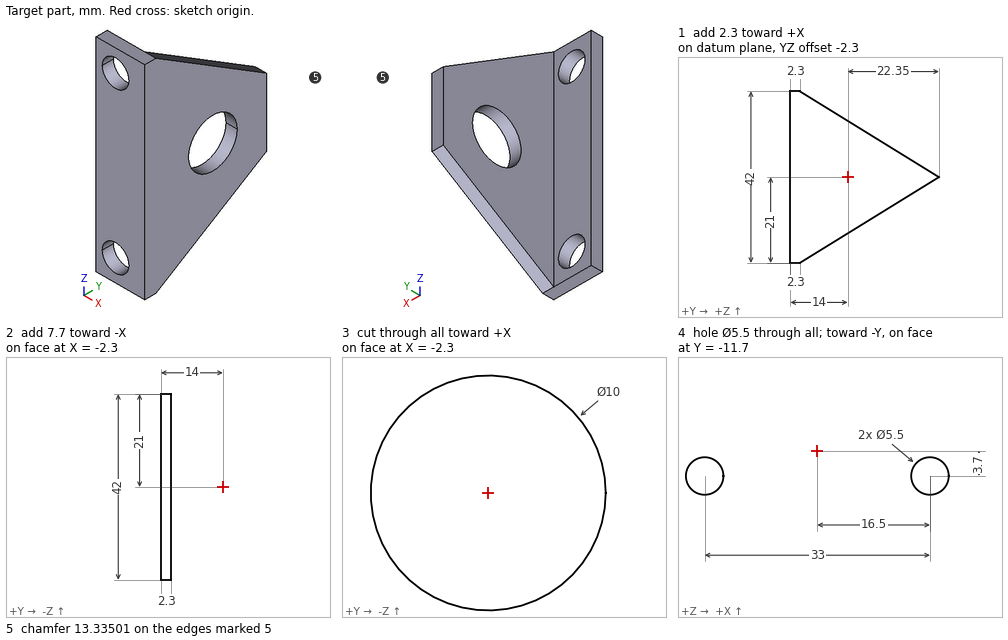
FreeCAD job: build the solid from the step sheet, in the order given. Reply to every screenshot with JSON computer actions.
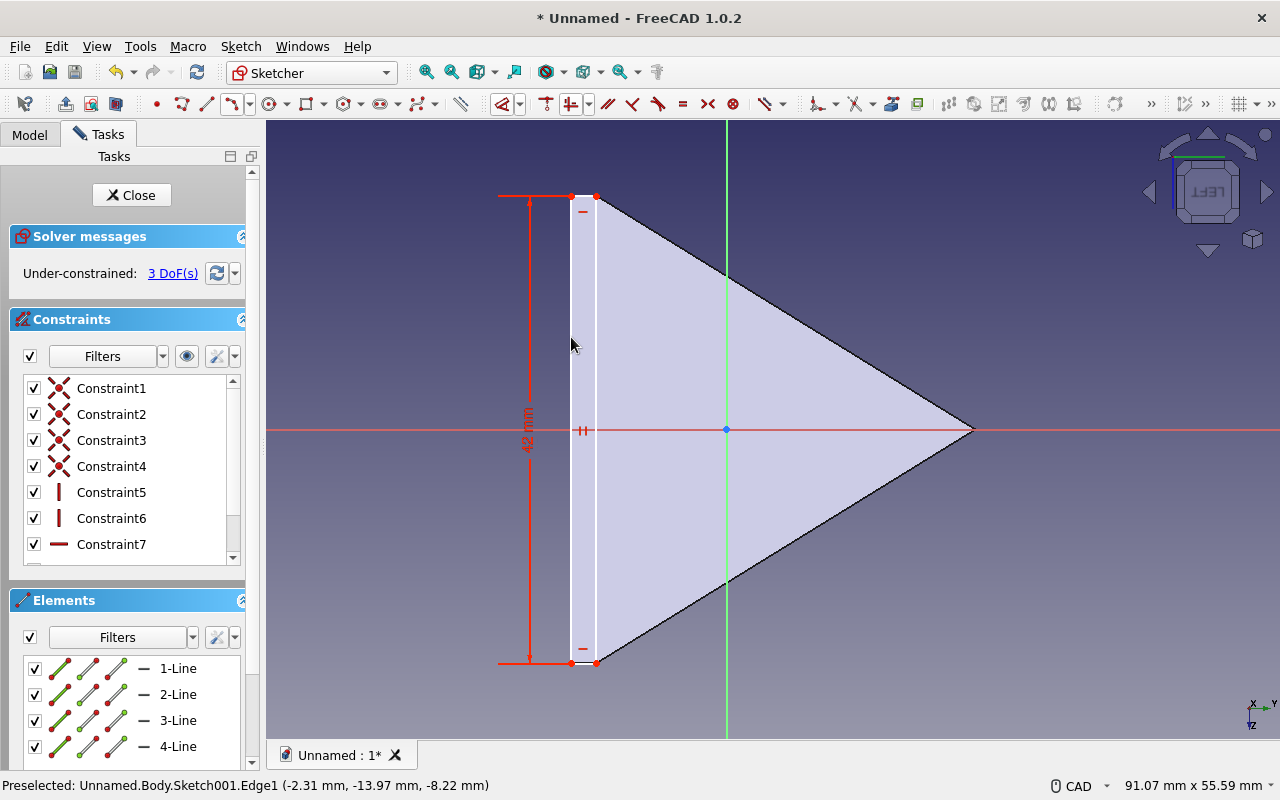
{"action": "scroll", "coordinate": [581, 664], "scroll_direction": "up", "scroll_amount": 3}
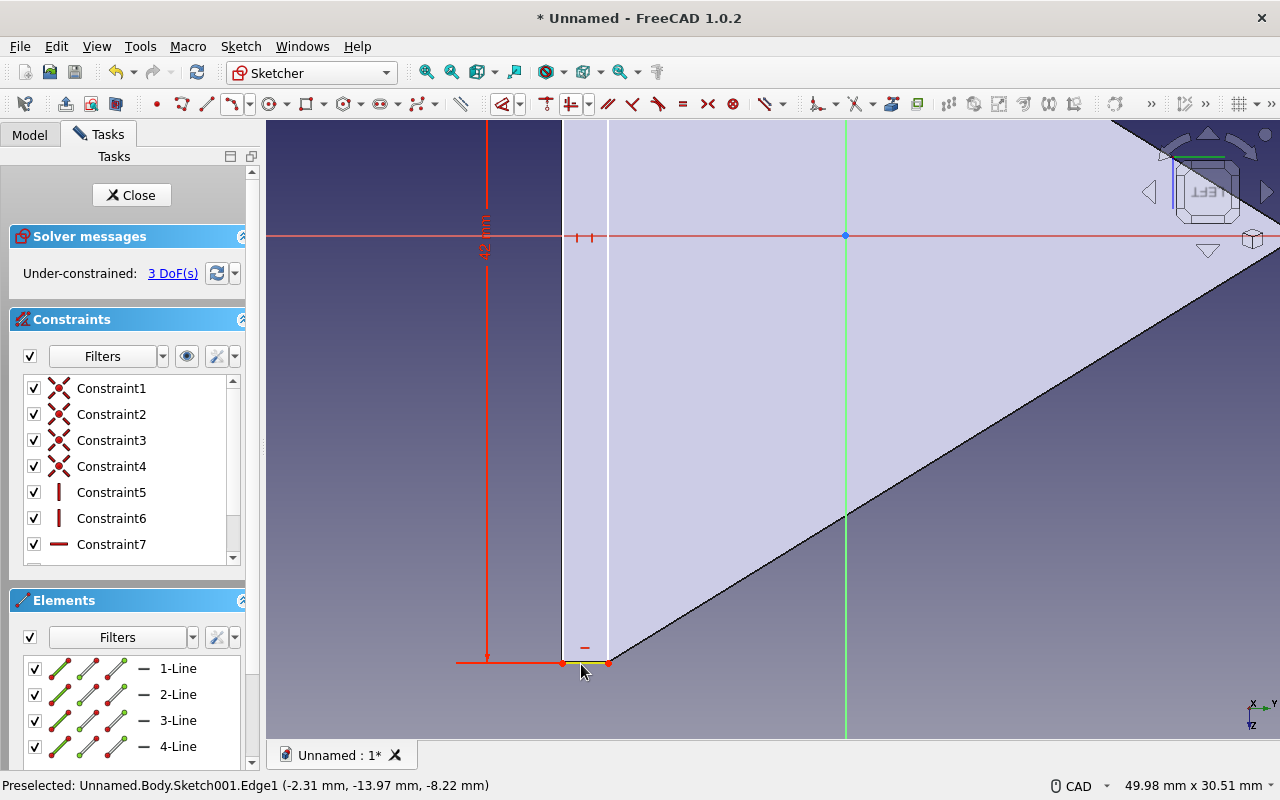
{"action": "left_click", "coordinate": [581, 663]}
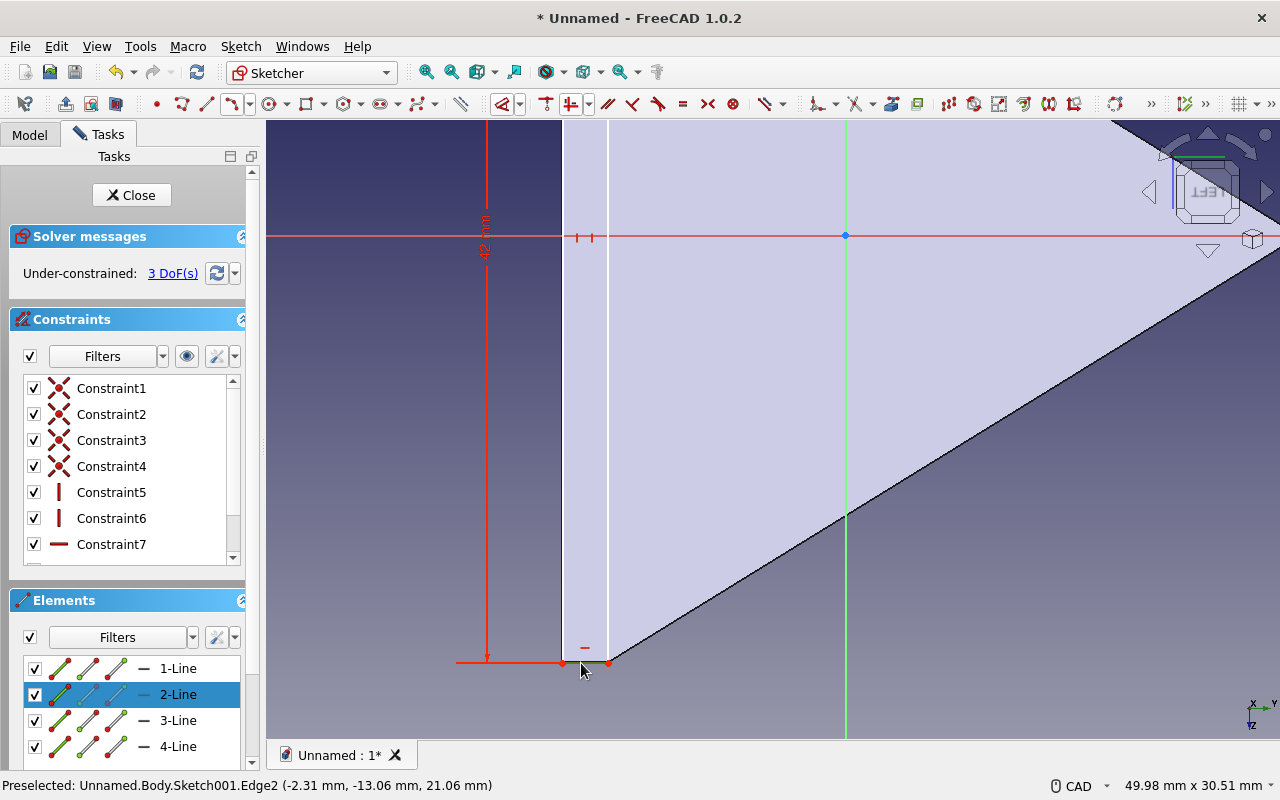
{"action": "left_click", "coordinate": [520, 104]}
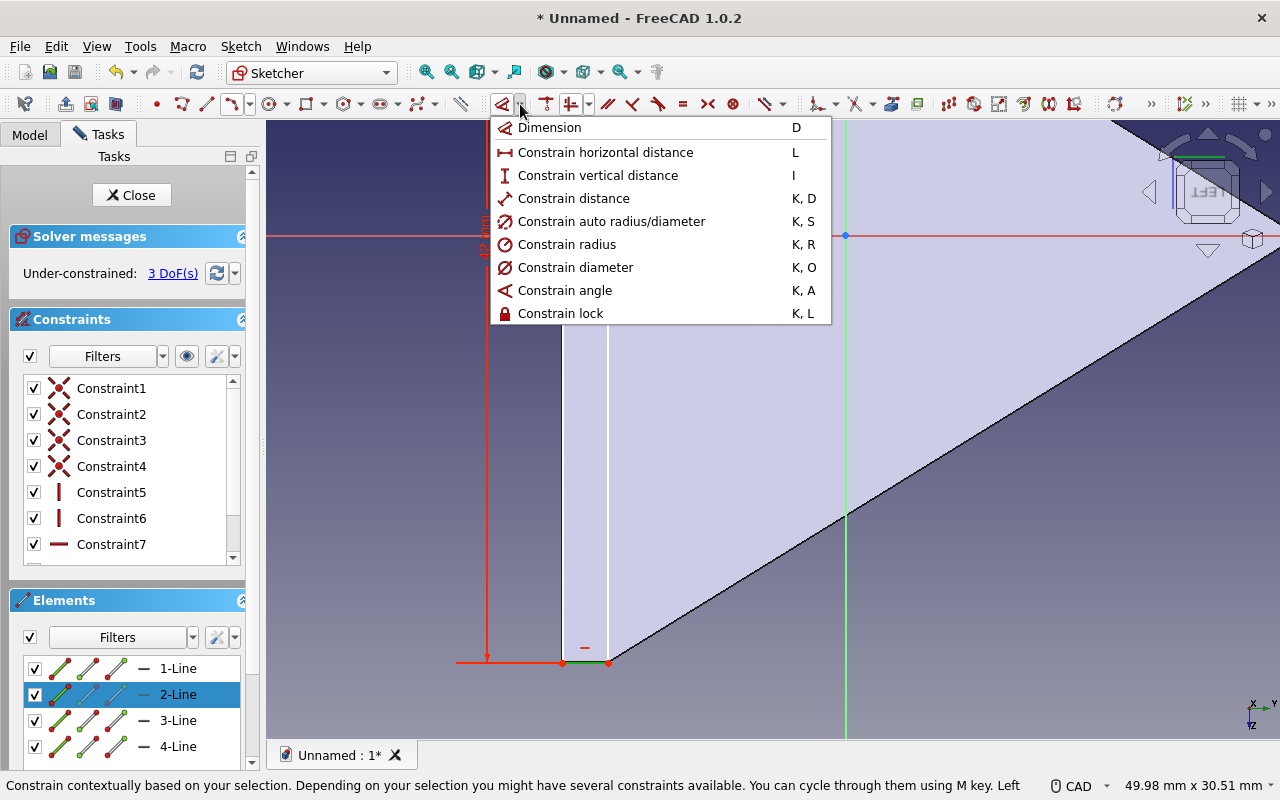
{"action": "left_click", "coordinate": [661, 152]}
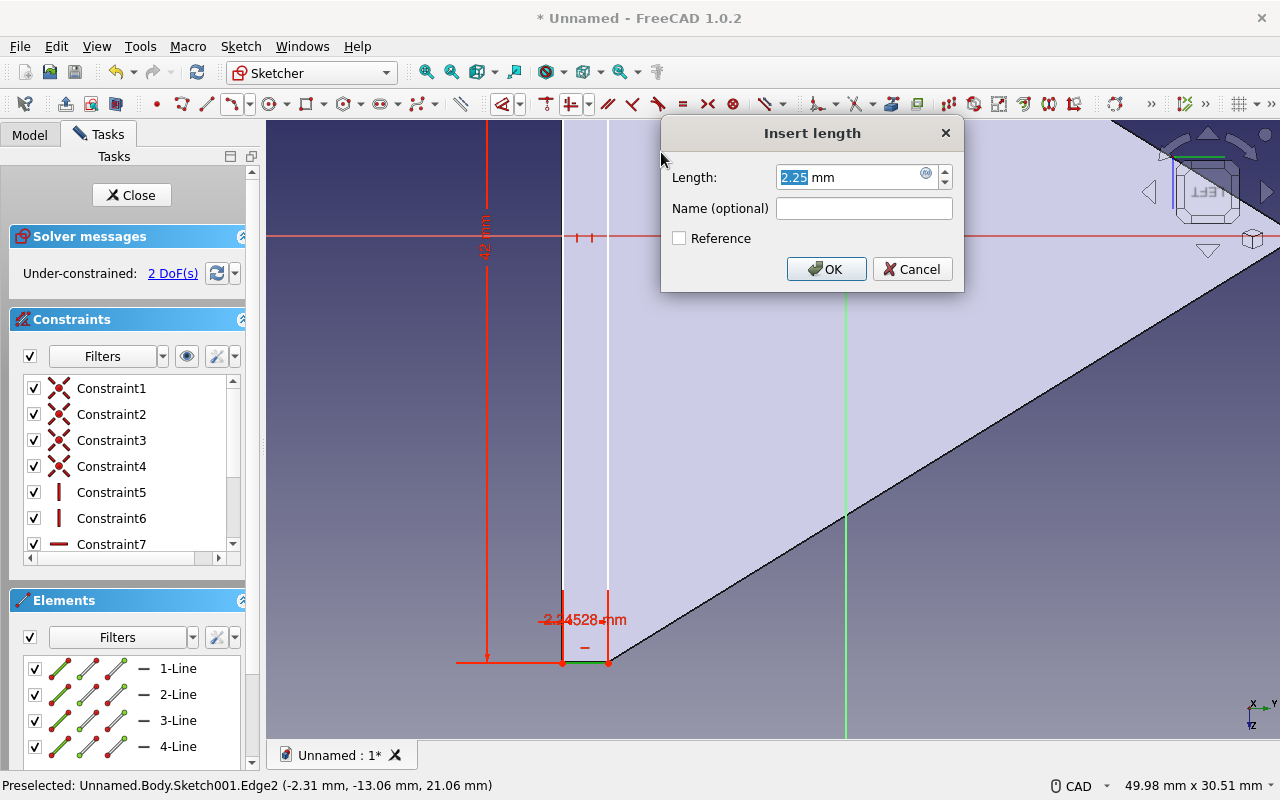
{"action": "type", "text": "2.3"}
{"action": "key", "text": "Return"}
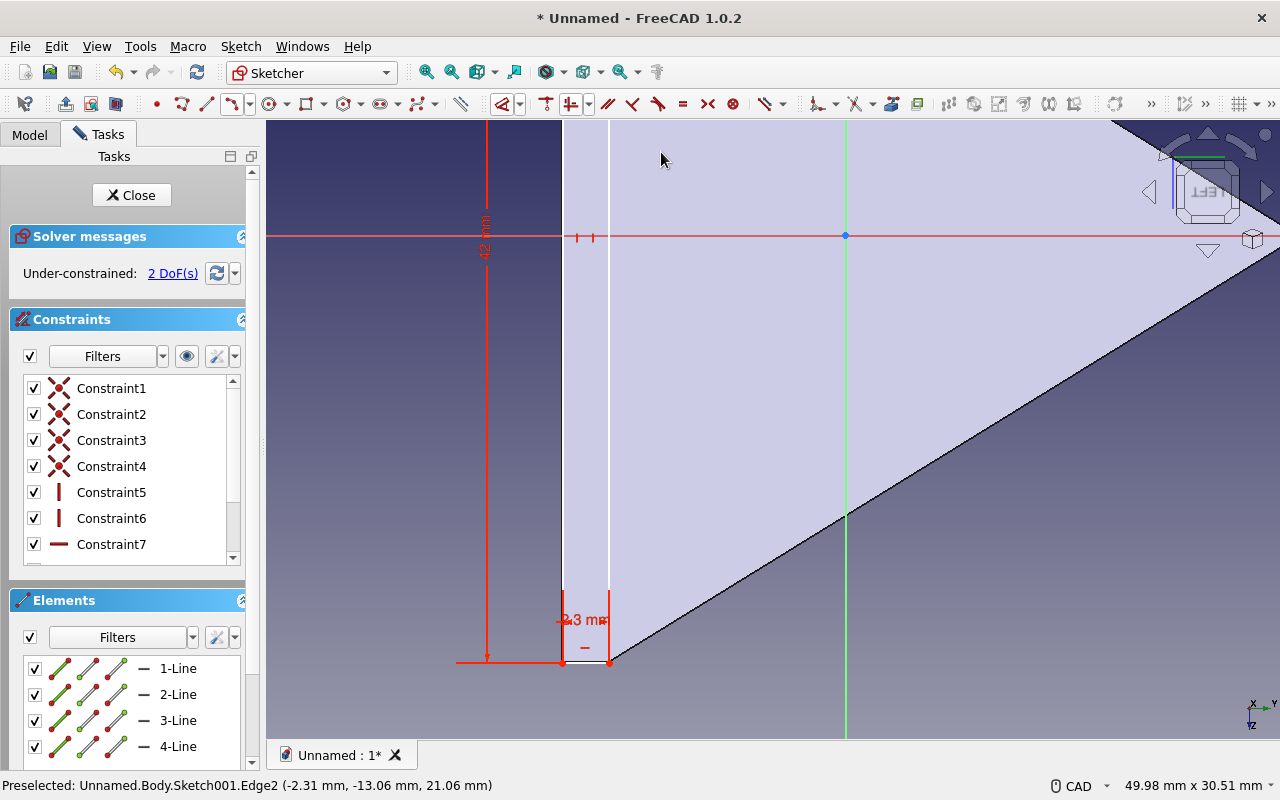
{"action": "scroll", "coordinate": [705, 587], "scroll_direction": "down", "scroll_amount": 4}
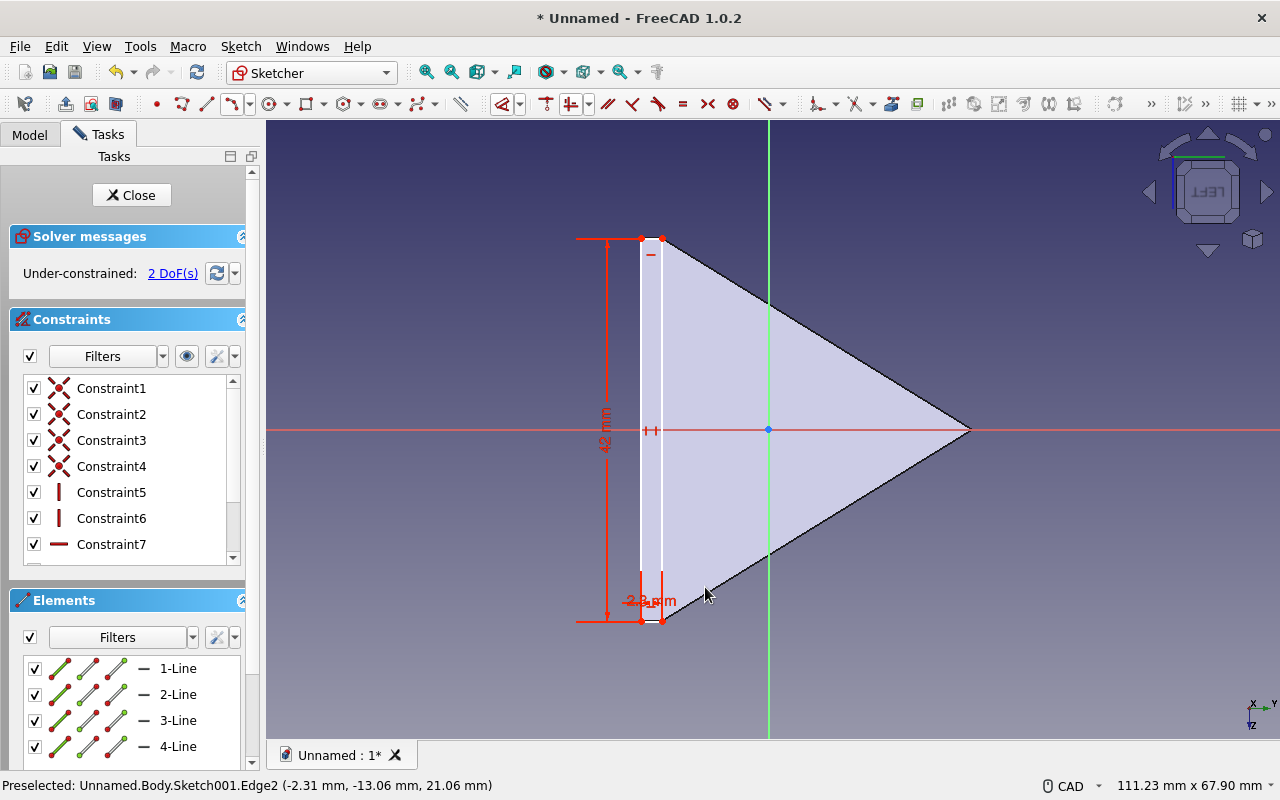
{"action": "left_click", "coordinate": [641, 239]}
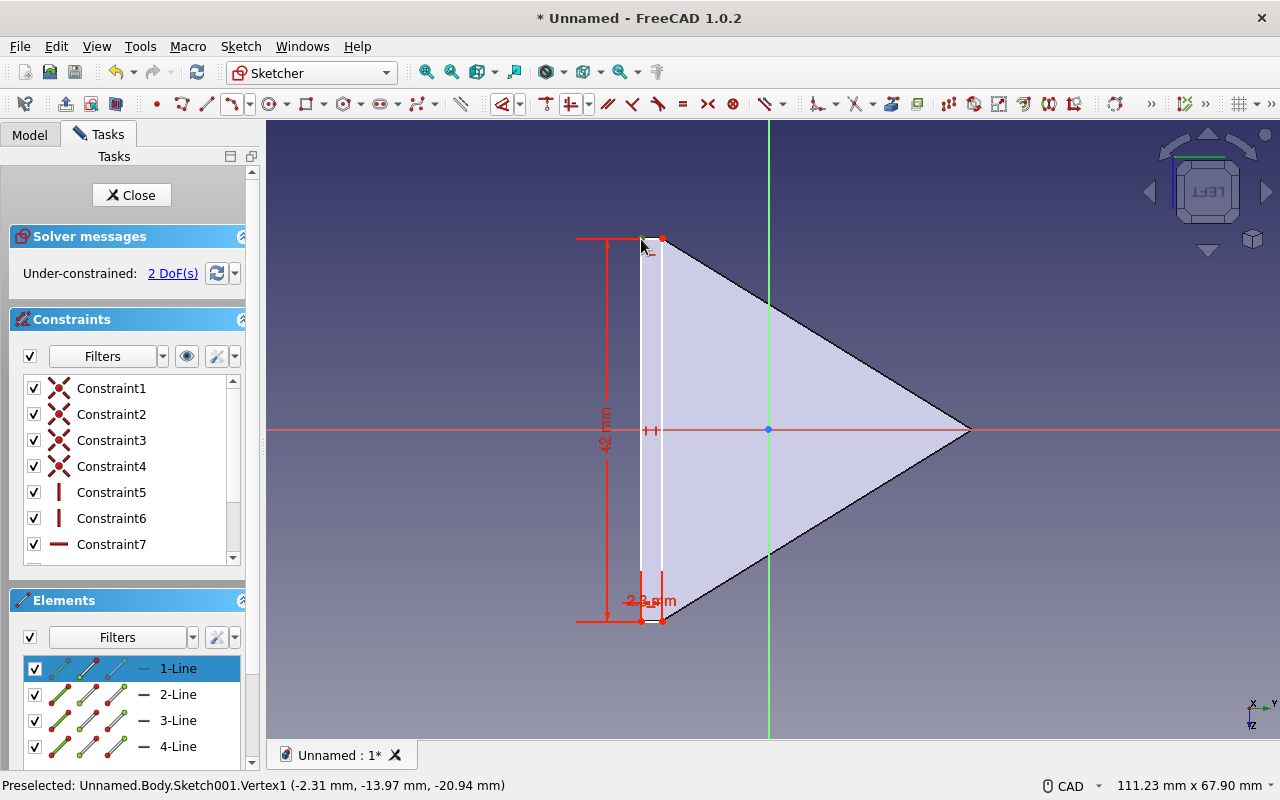
{"action": "key", "text": "l"}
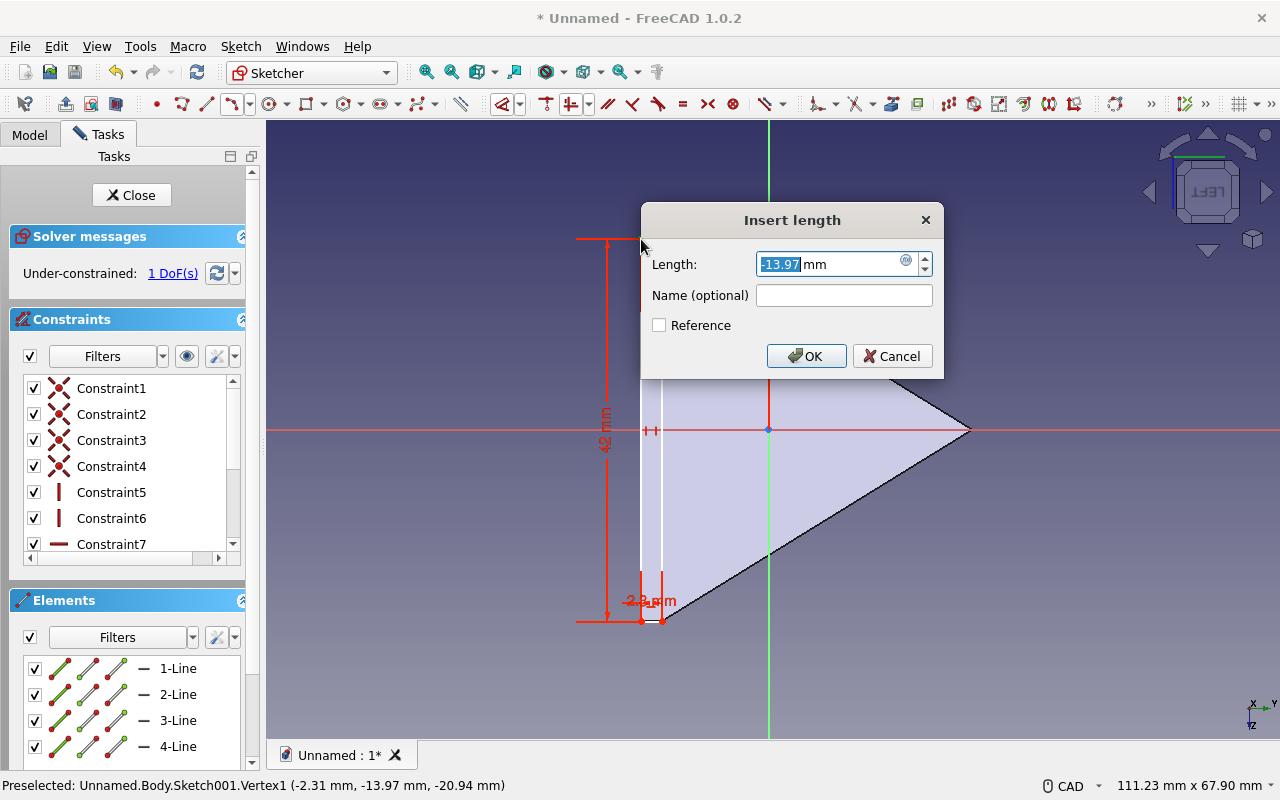
{"action": "type", "text": "-14"}
{"action": "key", "text": "Return"}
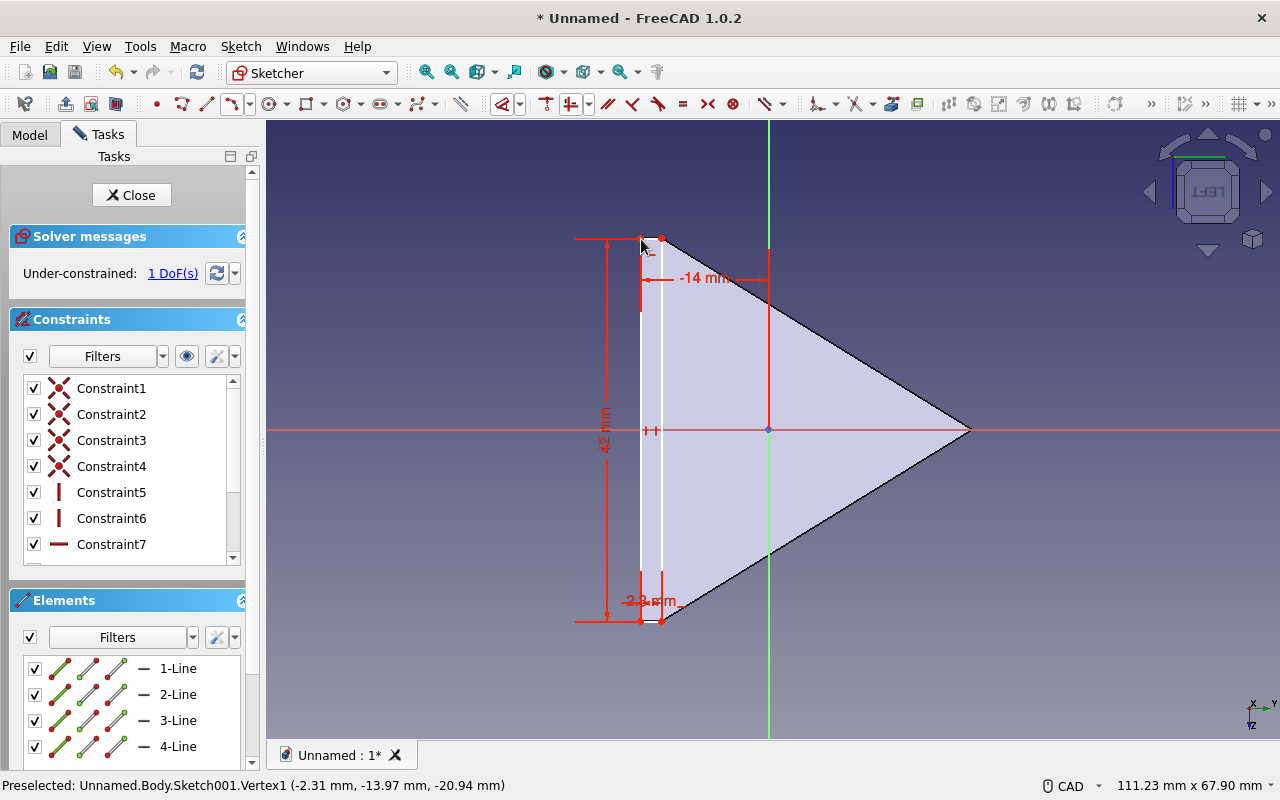
{"action": "left_click", "coordinate": [641, 239]}